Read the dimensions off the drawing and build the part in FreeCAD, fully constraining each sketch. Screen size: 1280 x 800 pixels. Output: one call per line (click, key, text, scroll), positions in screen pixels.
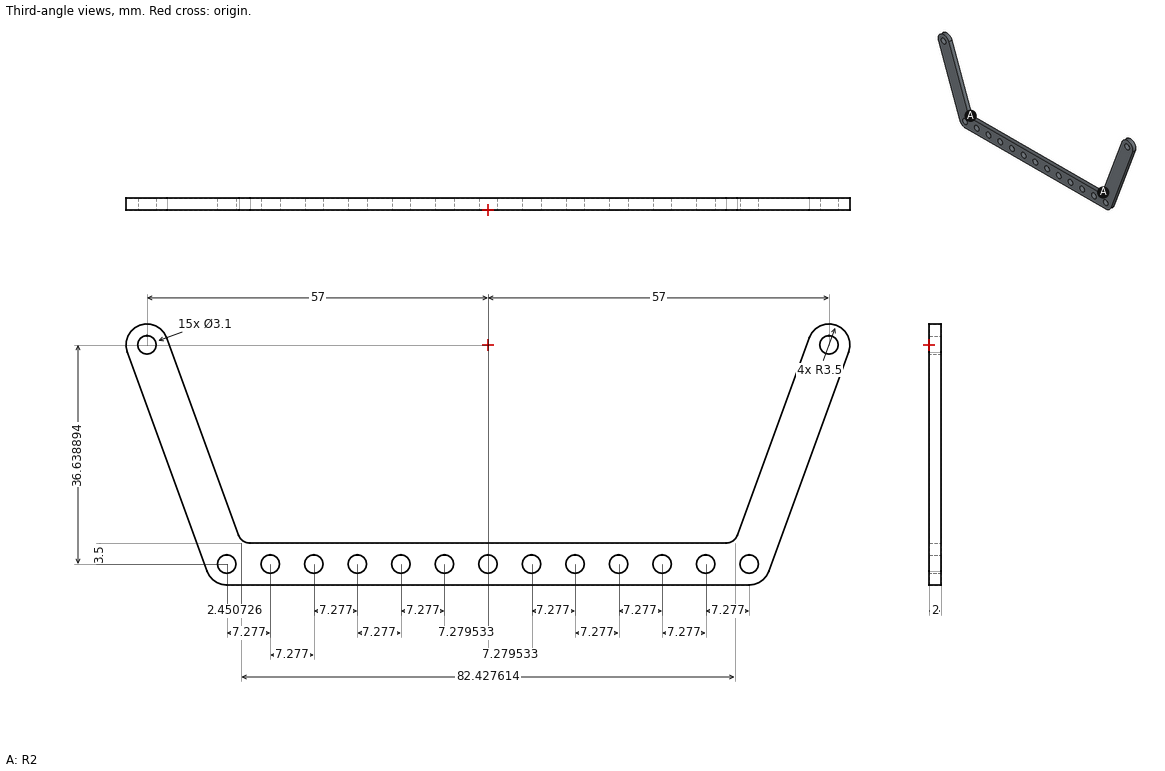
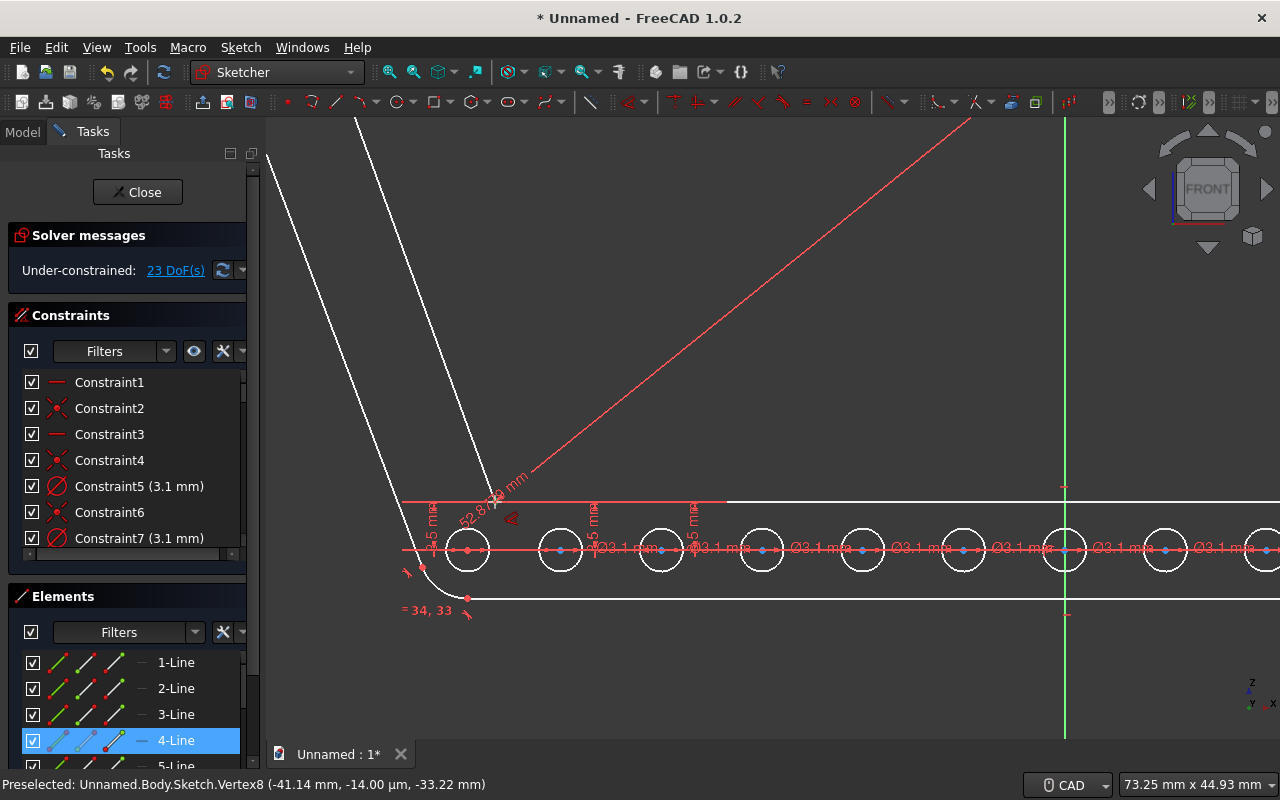
click(762, 550)
click(796, 526)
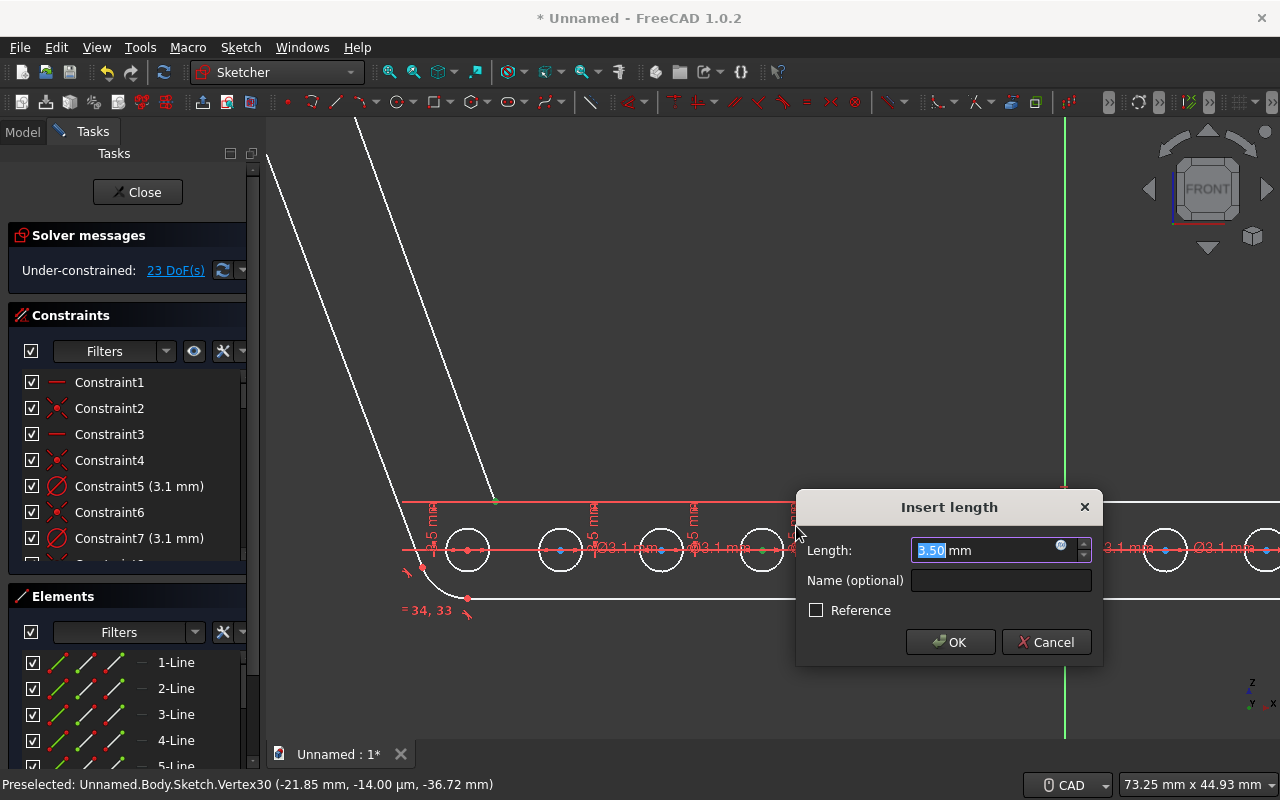
text(3.5)
key(Return)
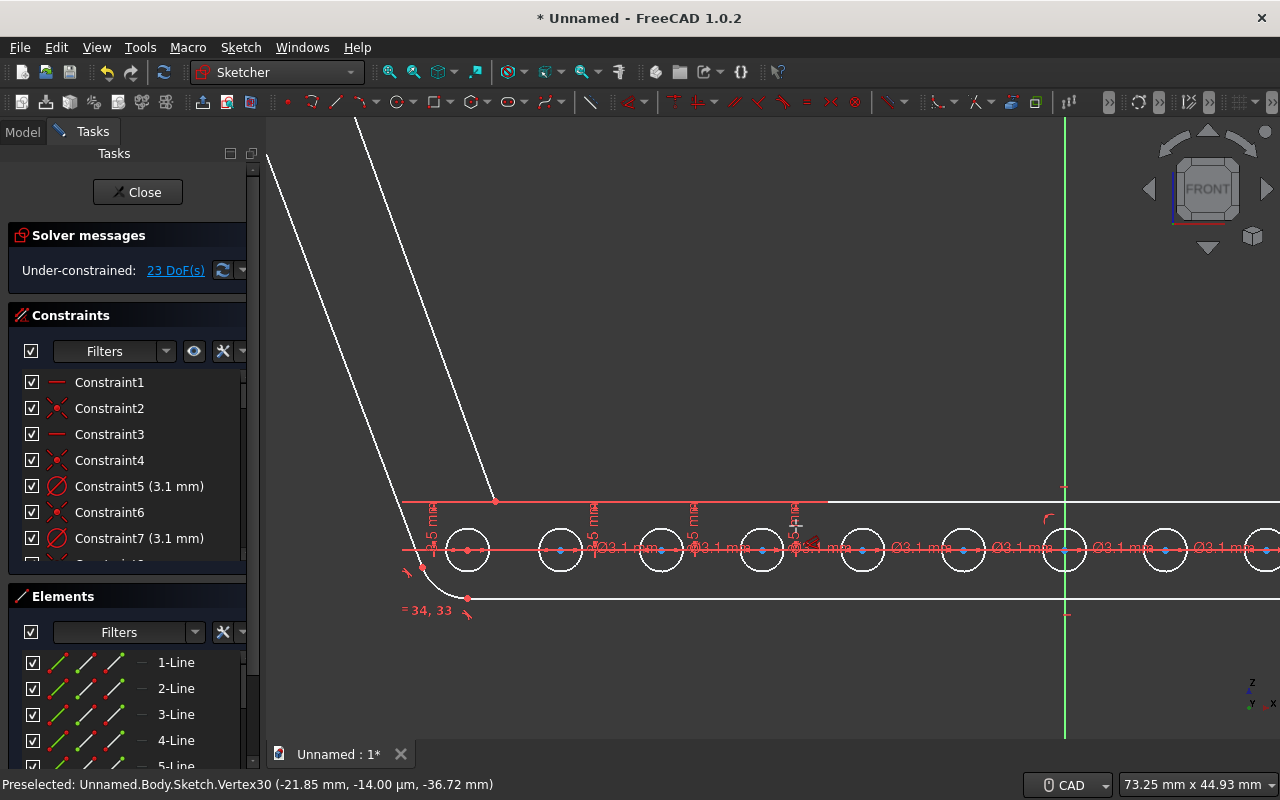
click(495, 502)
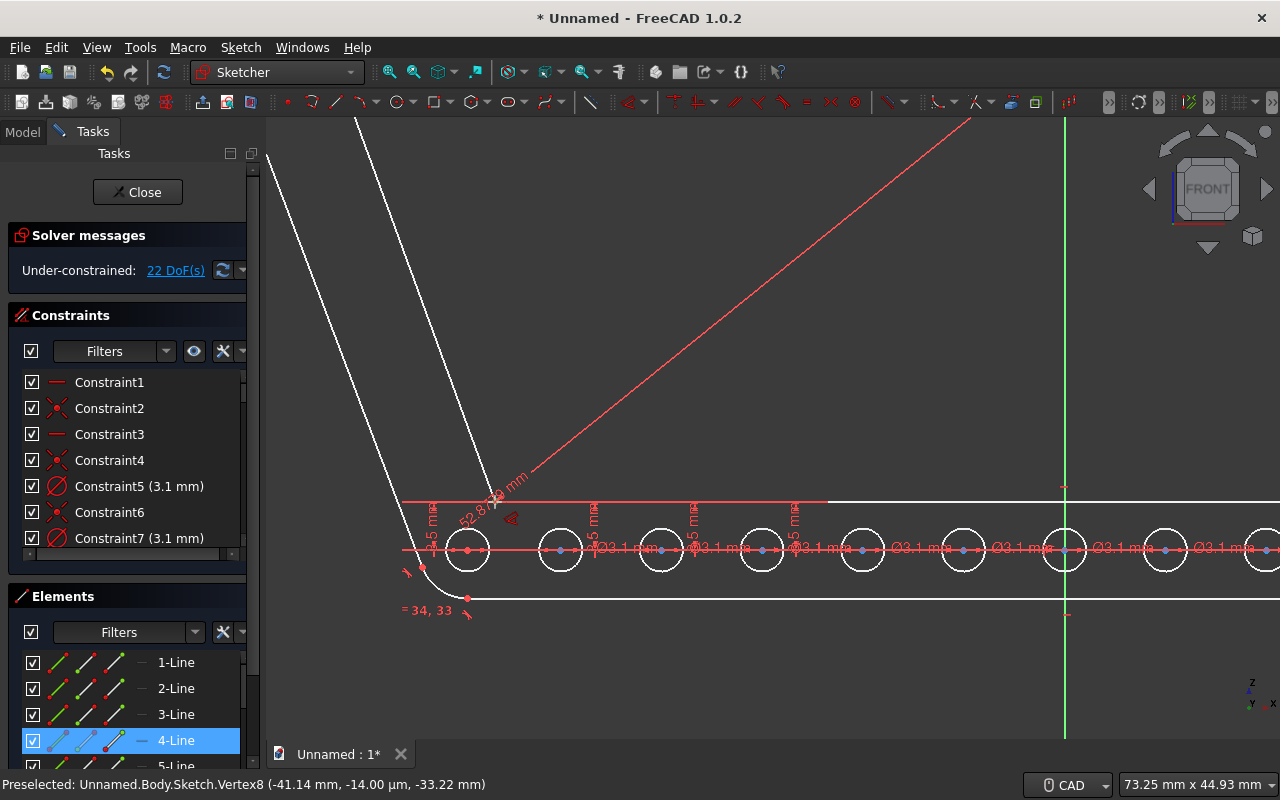
click(863, 550)
click(897, 526)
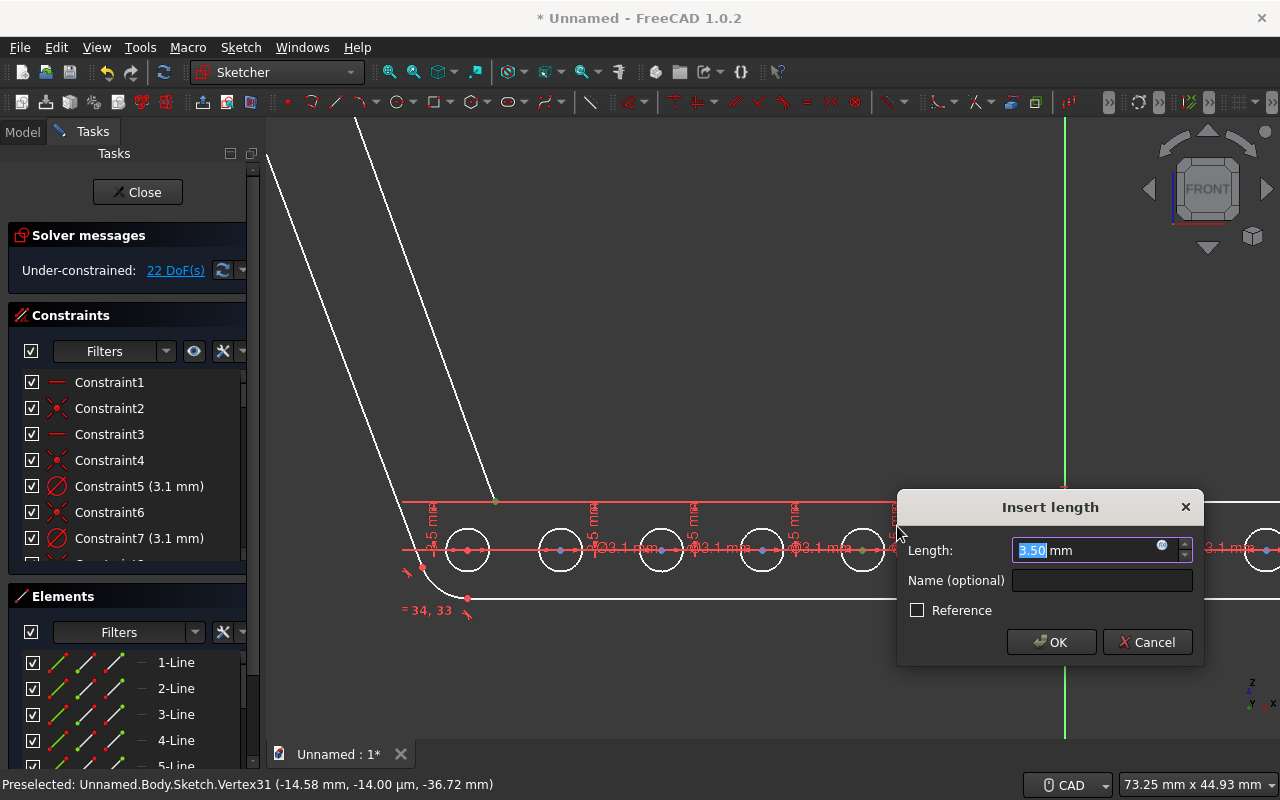
text(3.5)
key(Return)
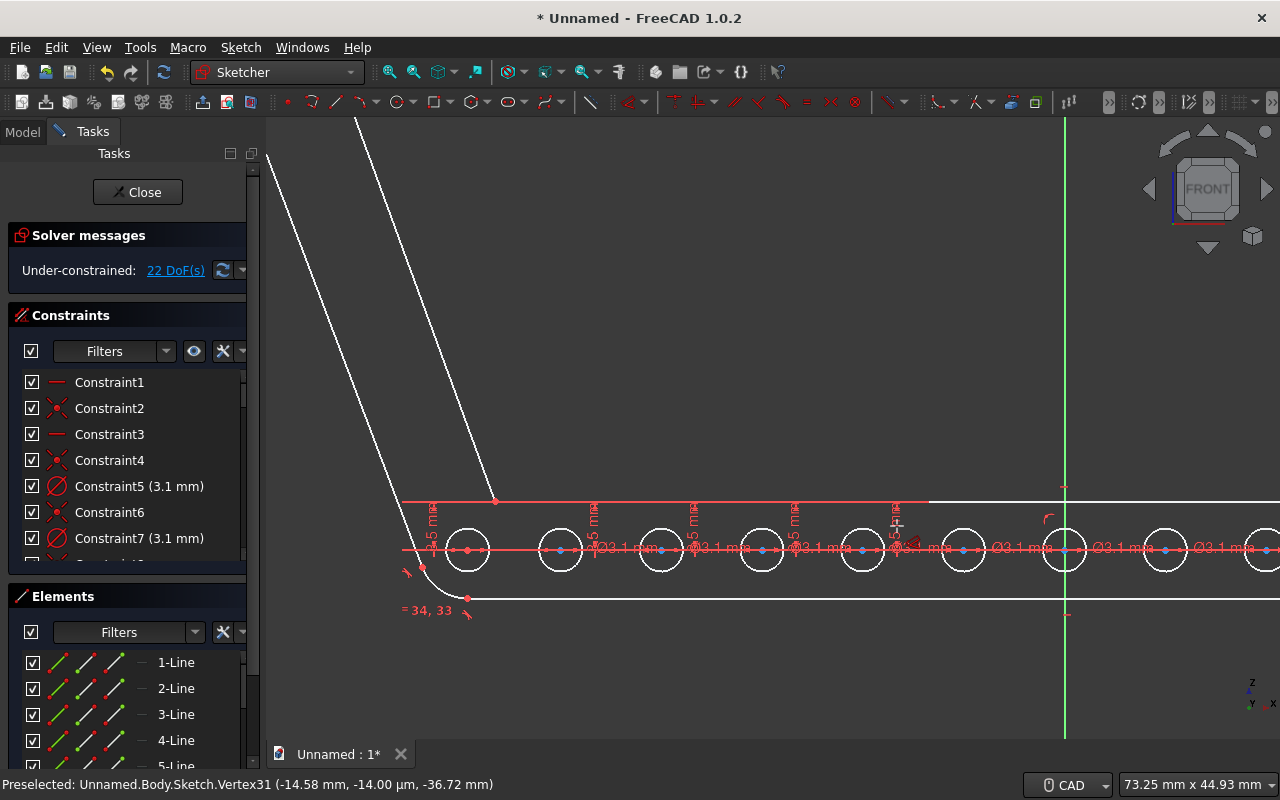
click(495, 502)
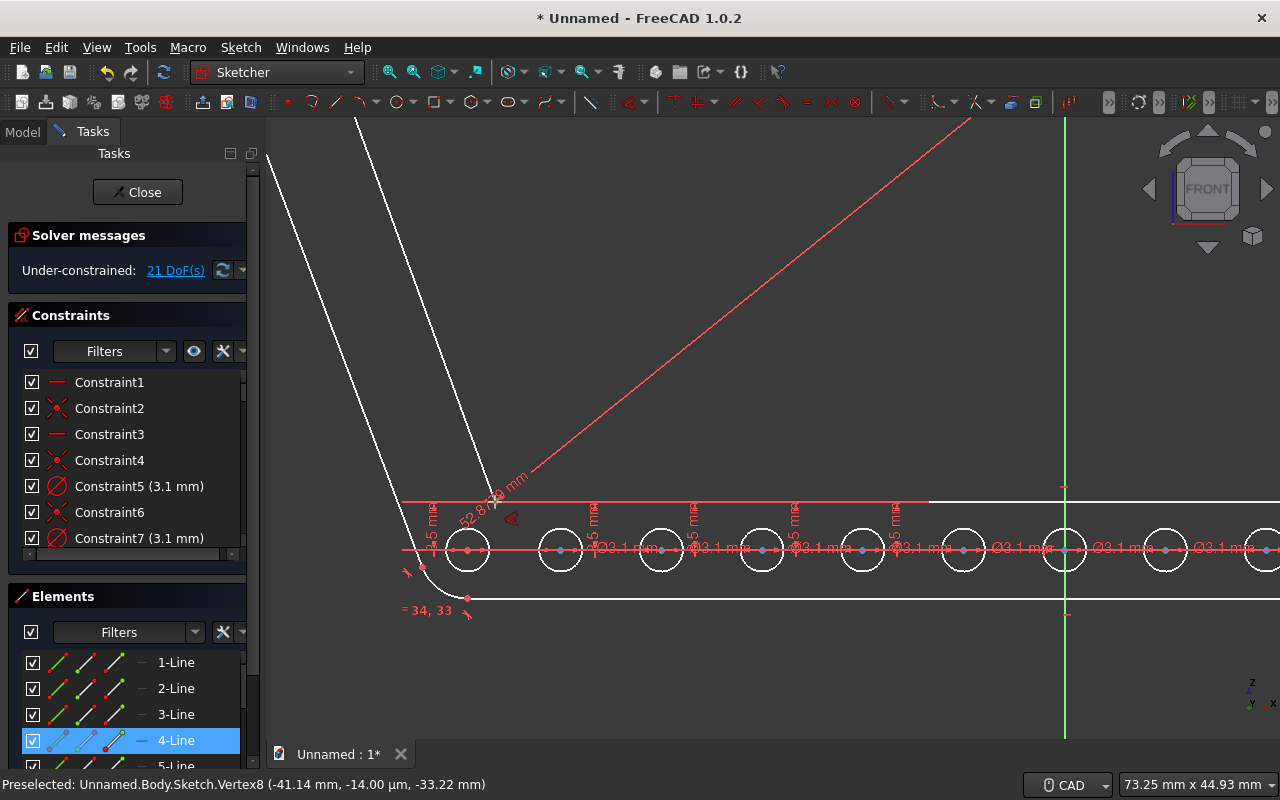
click(964, 550)
click(998, 526)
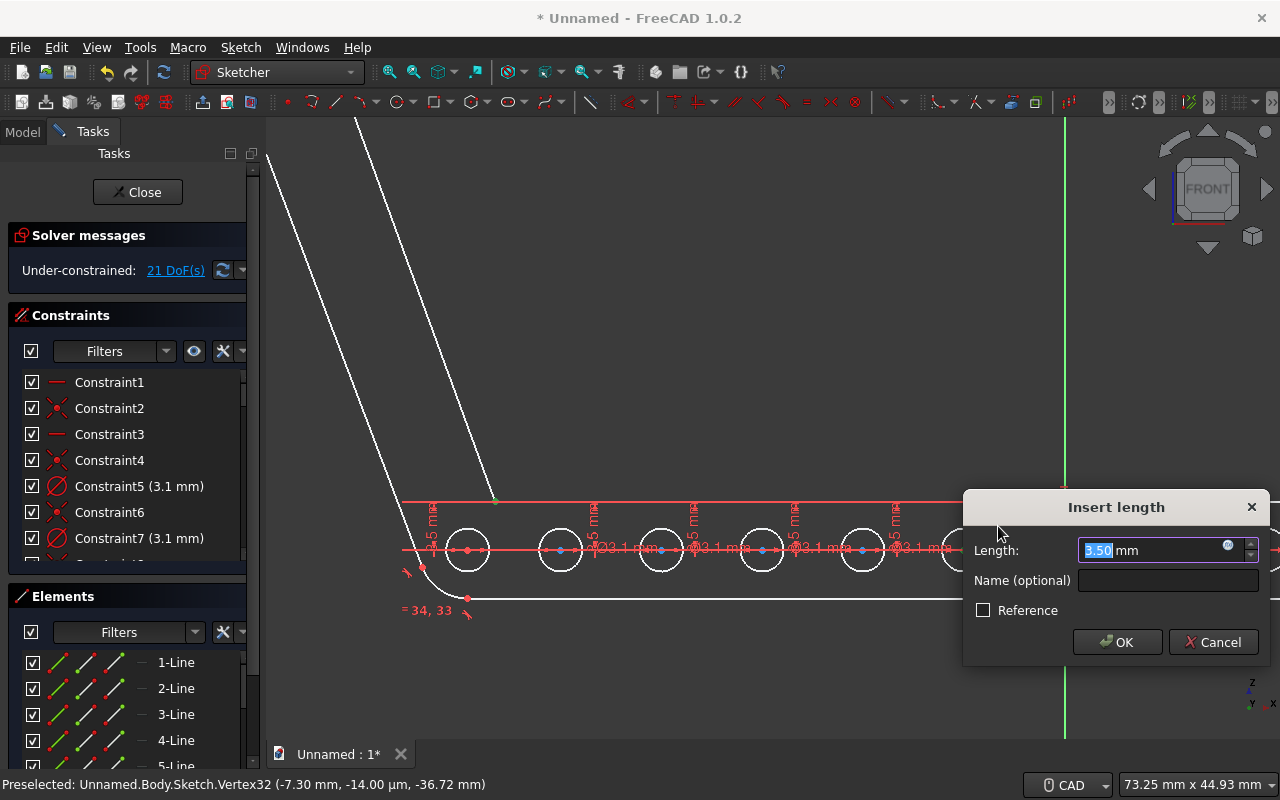
text(3.5)
key(Return)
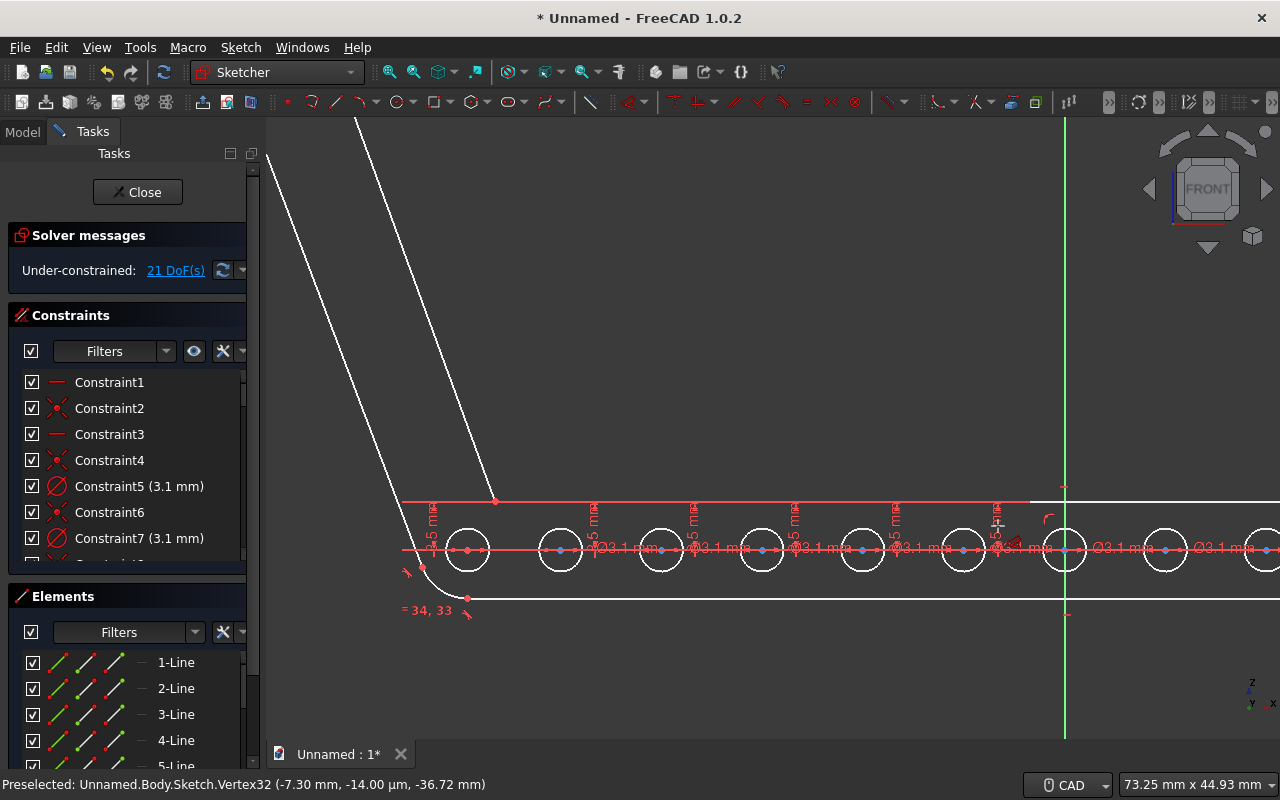
click(495, 502)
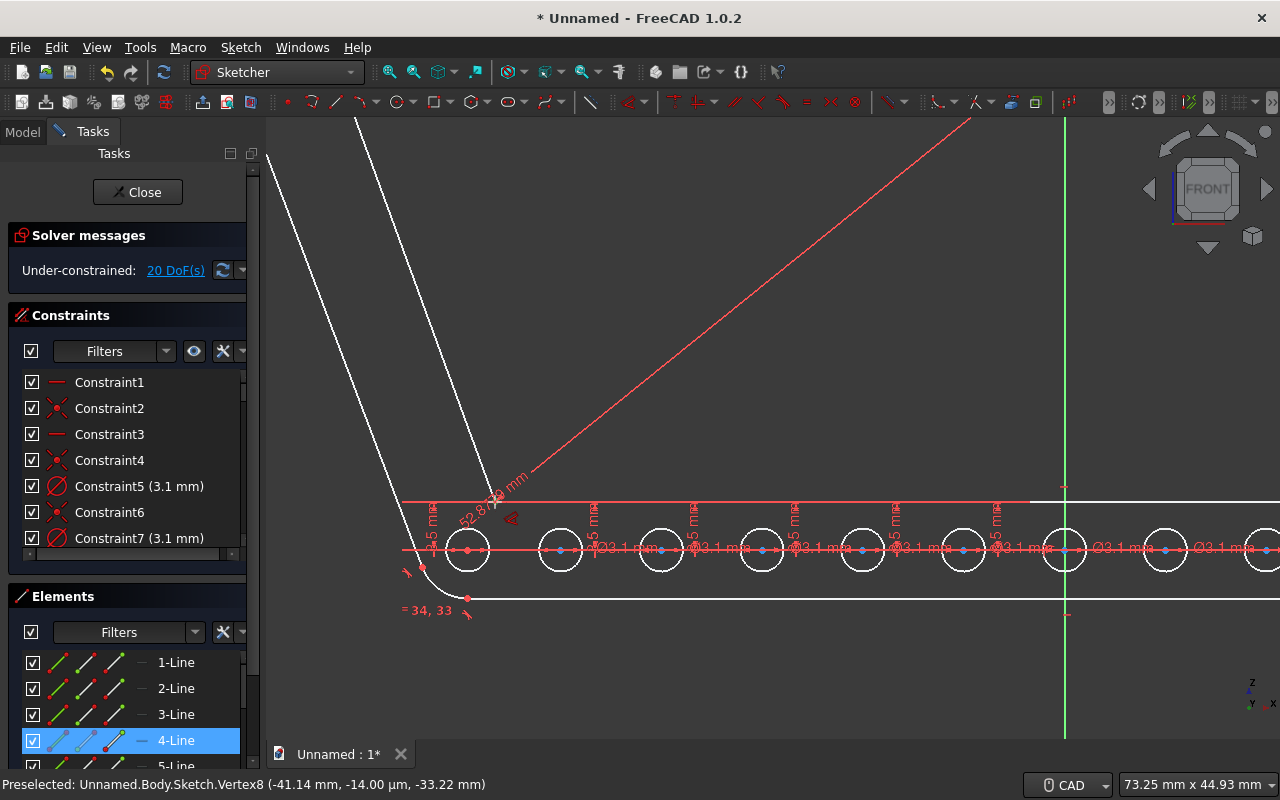
click(1065, 550)
click(1099, 526)